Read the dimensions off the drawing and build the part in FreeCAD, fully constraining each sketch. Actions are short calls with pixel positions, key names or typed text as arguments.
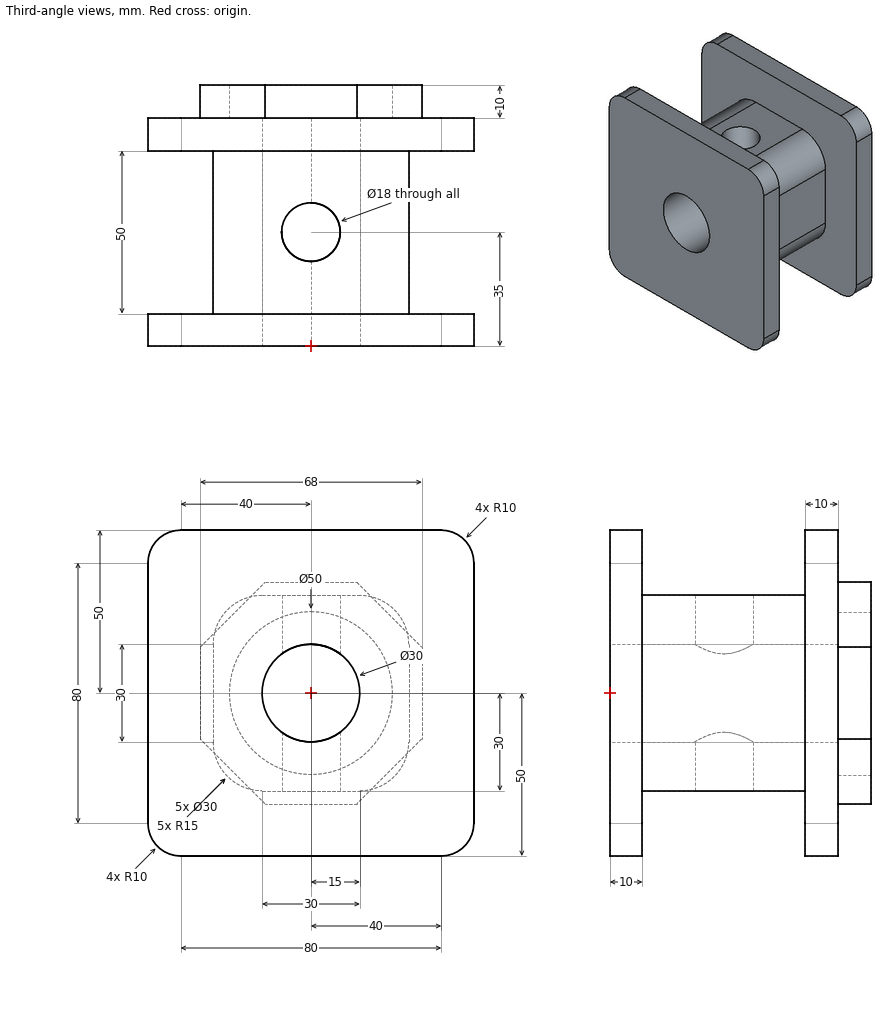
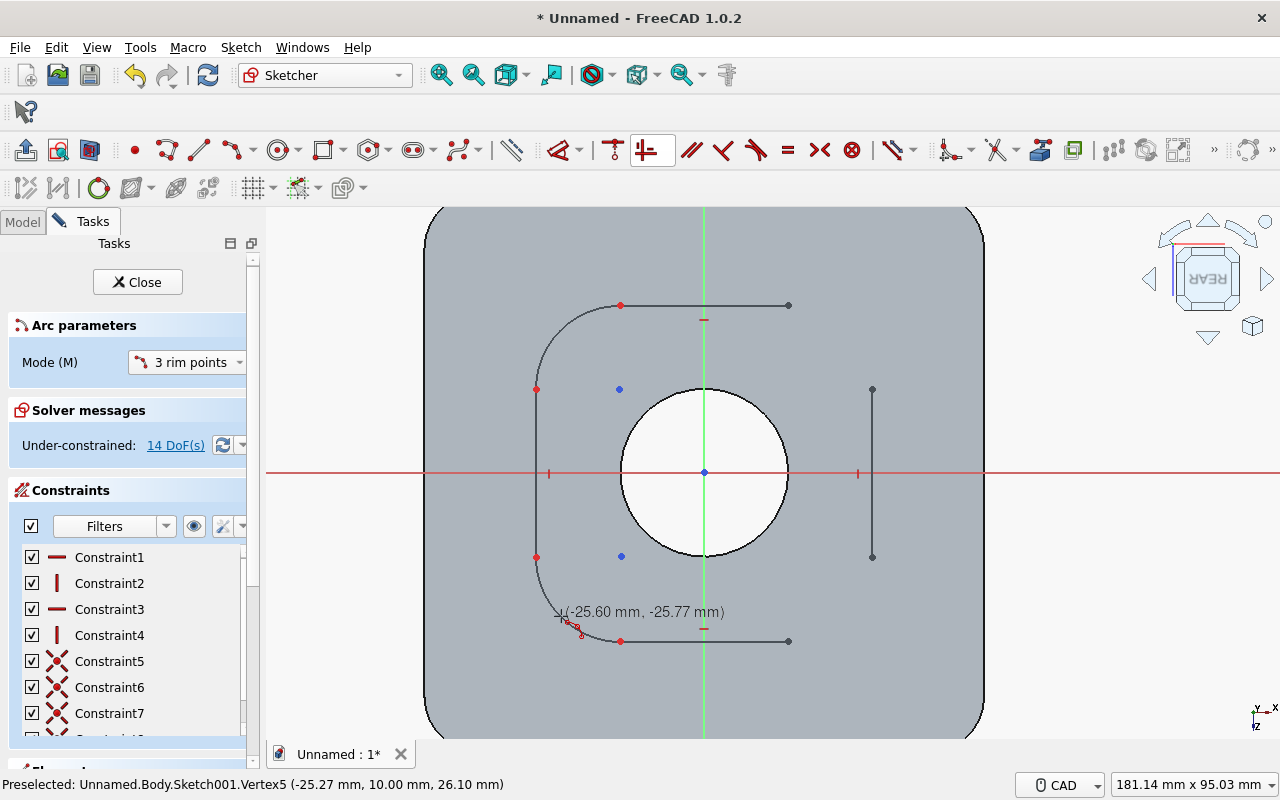
click(788, 642)
click(872, 558)
click(848, 616)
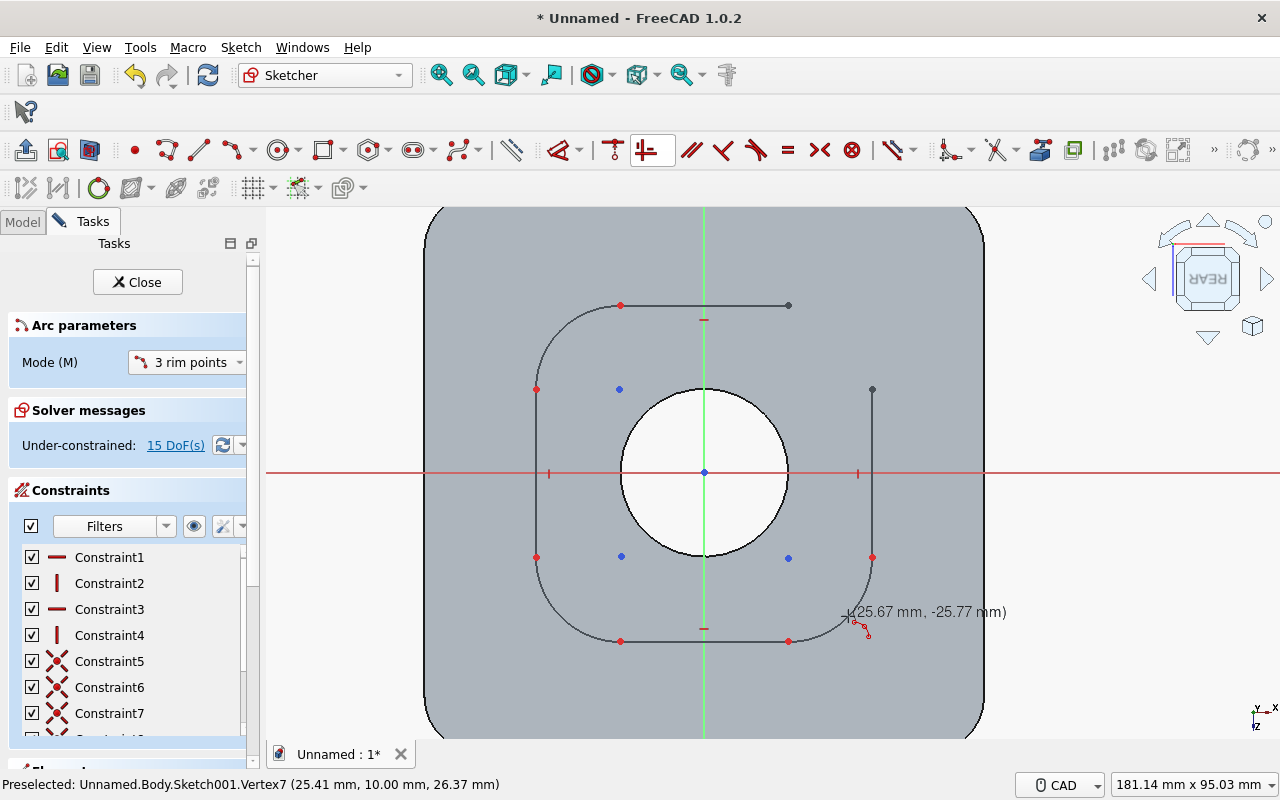
click(872, 390)
click(788, 306)
click(848, 329)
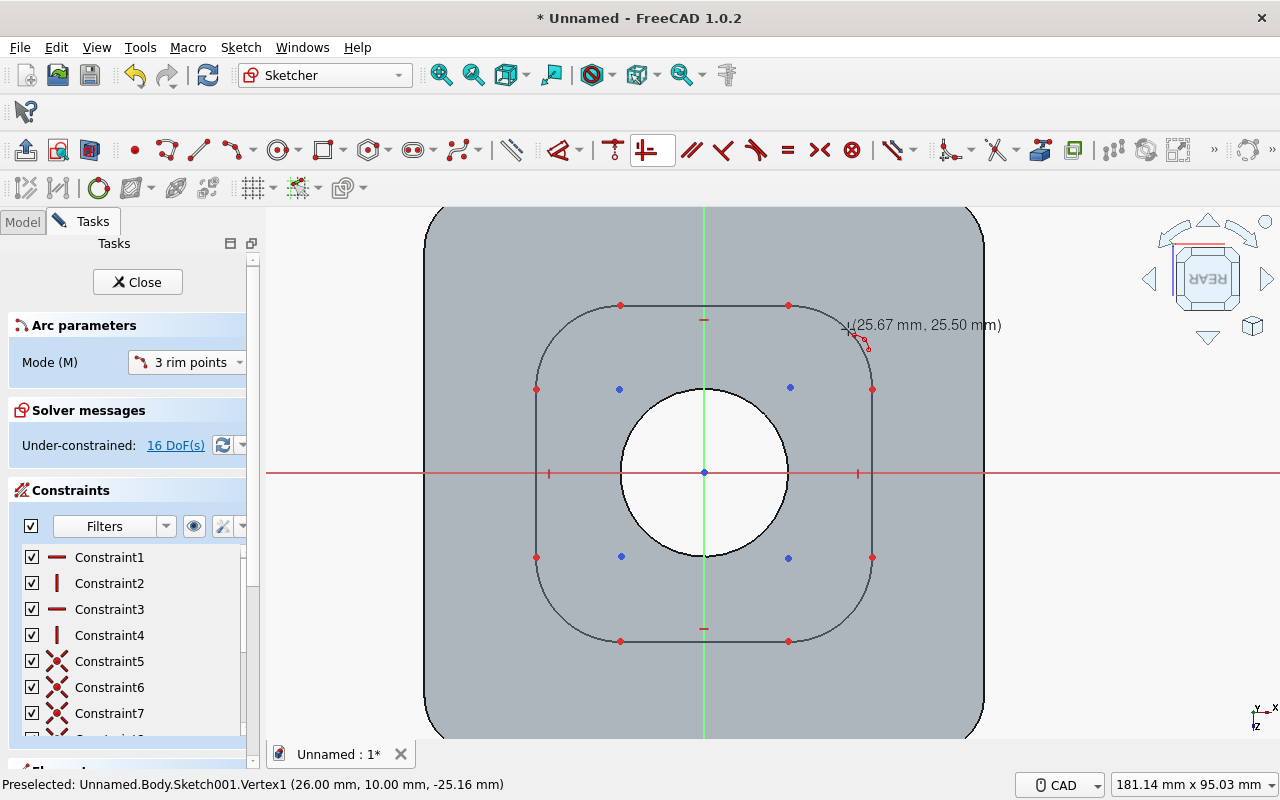
click(278, 150)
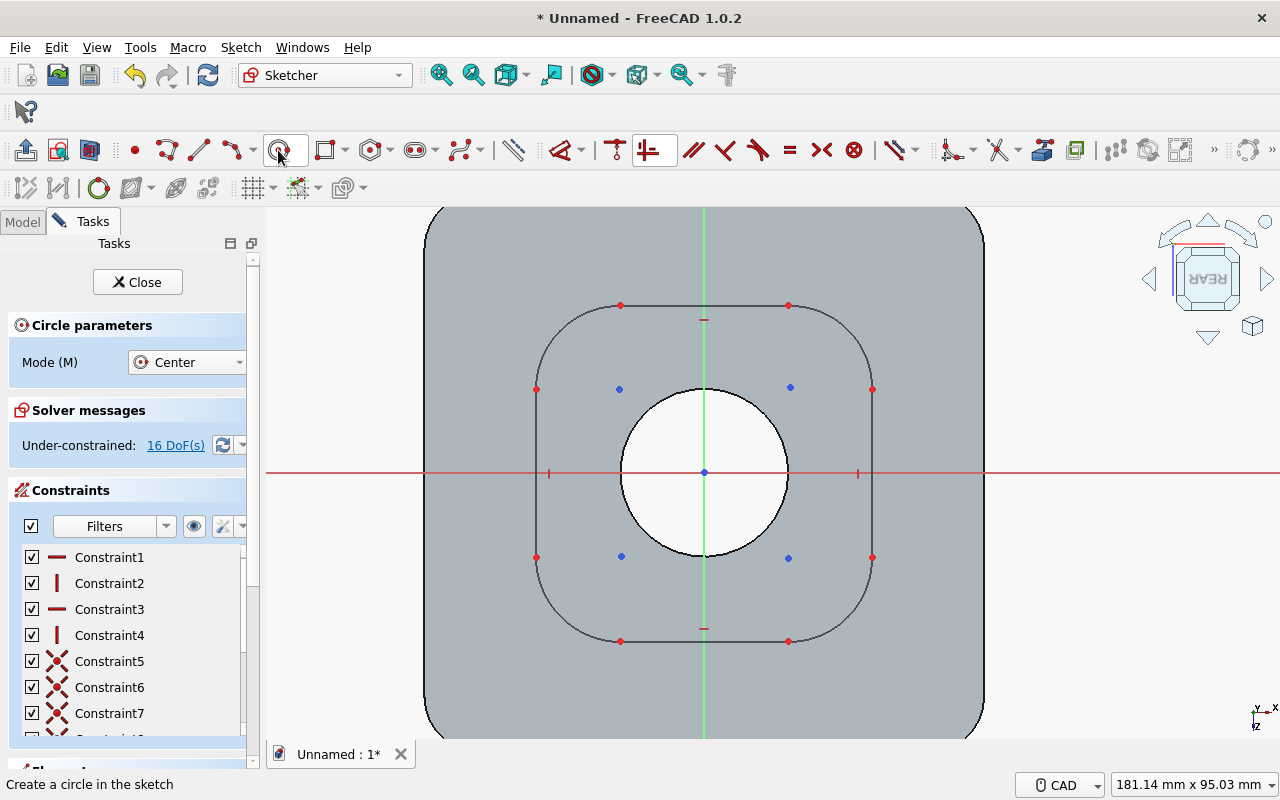
click(704, 473)
move(764, 413)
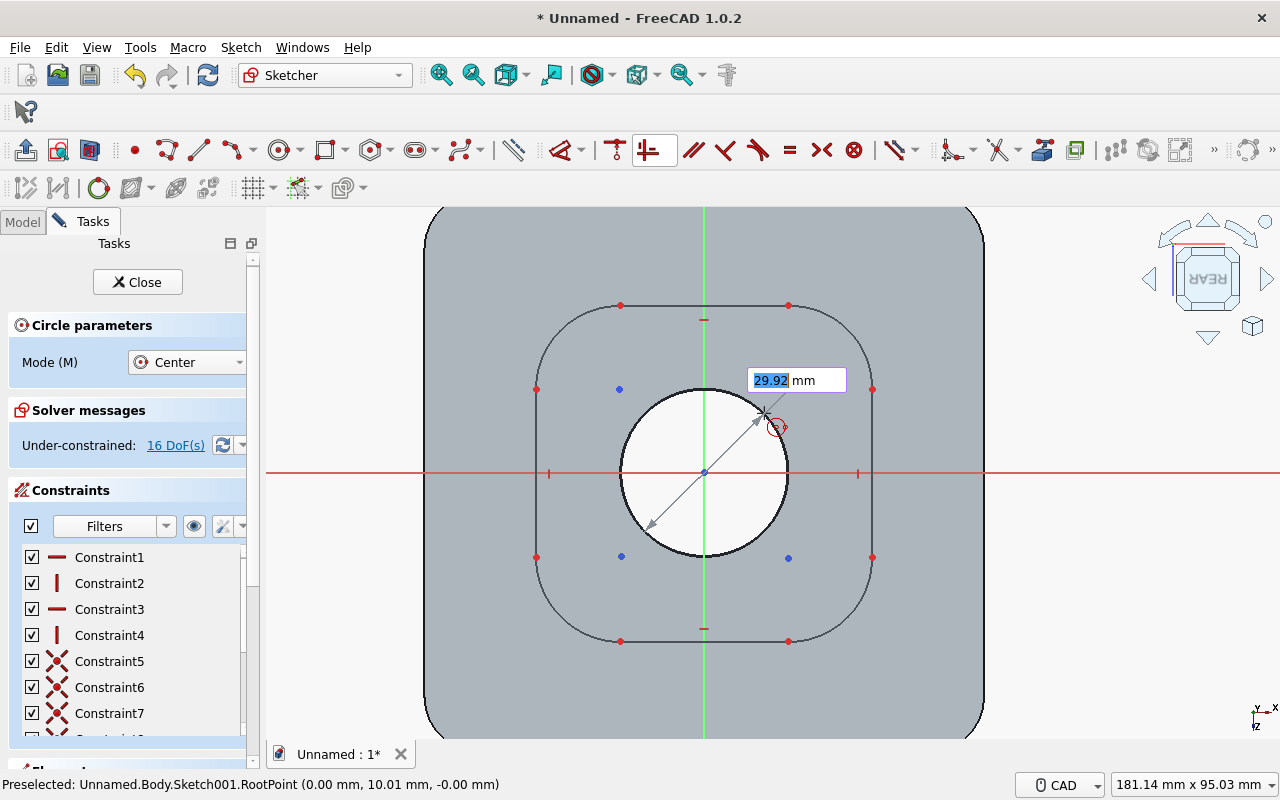
text(30)
key(Return)
key(Escape)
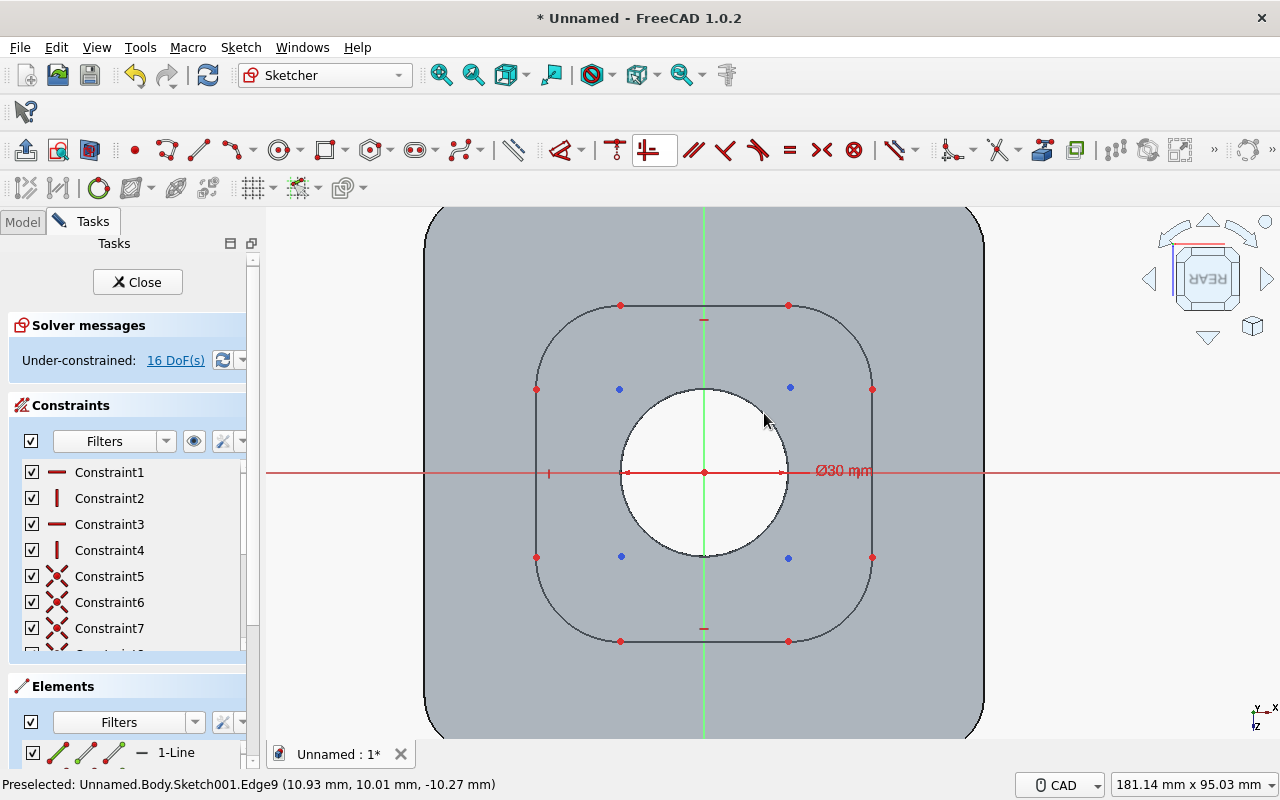
click(738, 306)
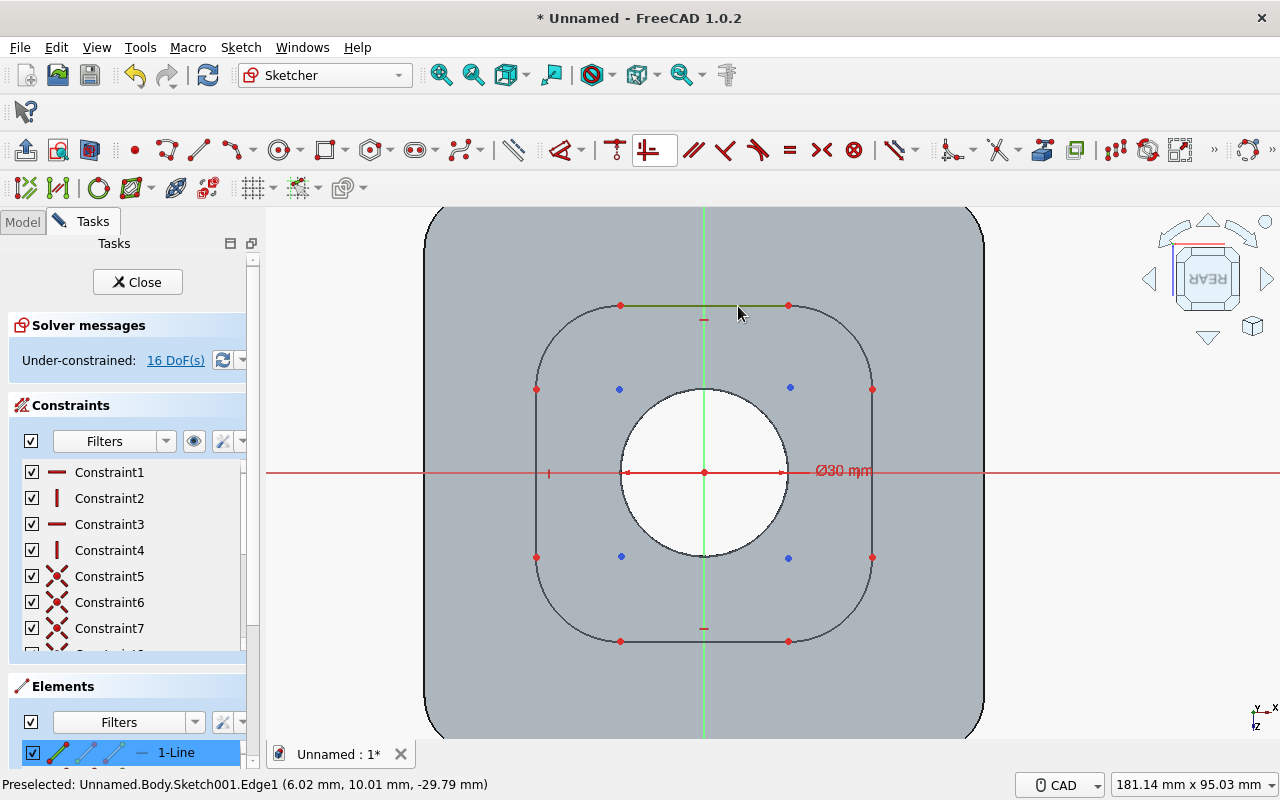
click(582, 315)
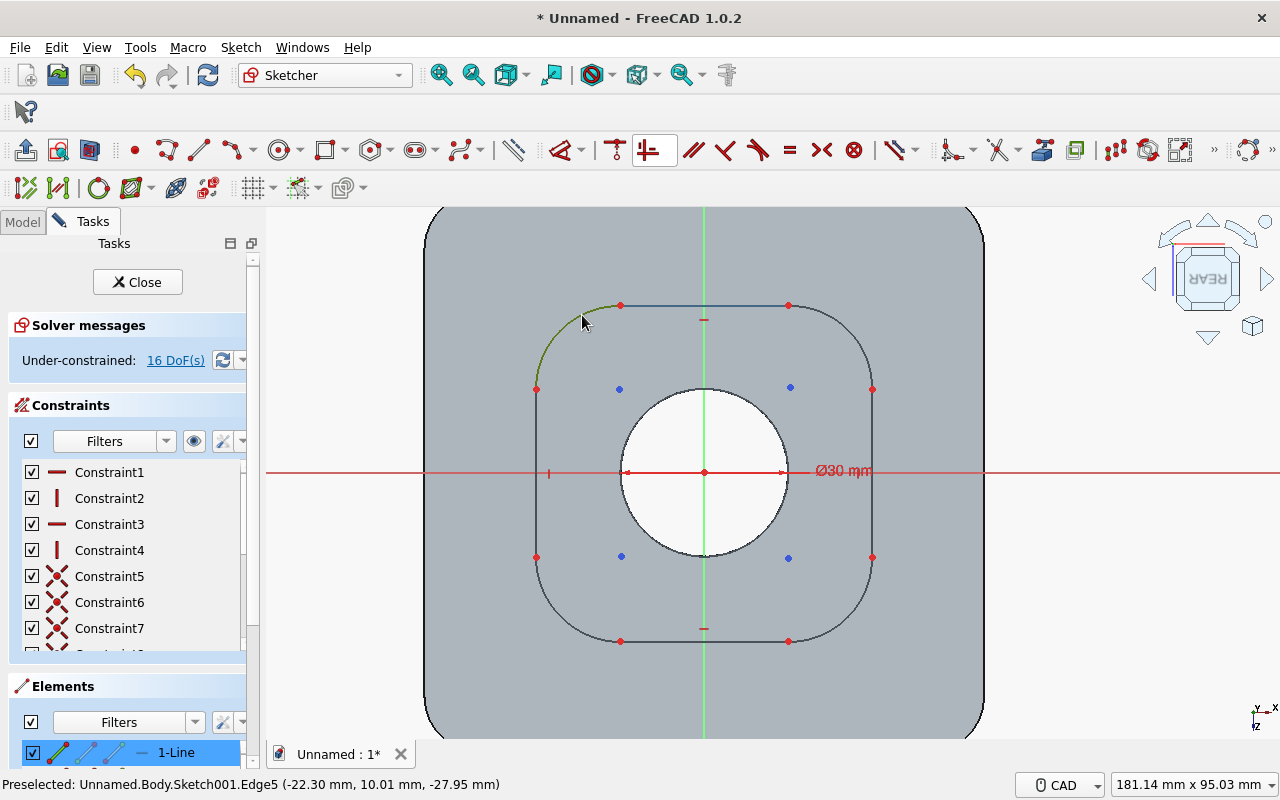
click(758, 150)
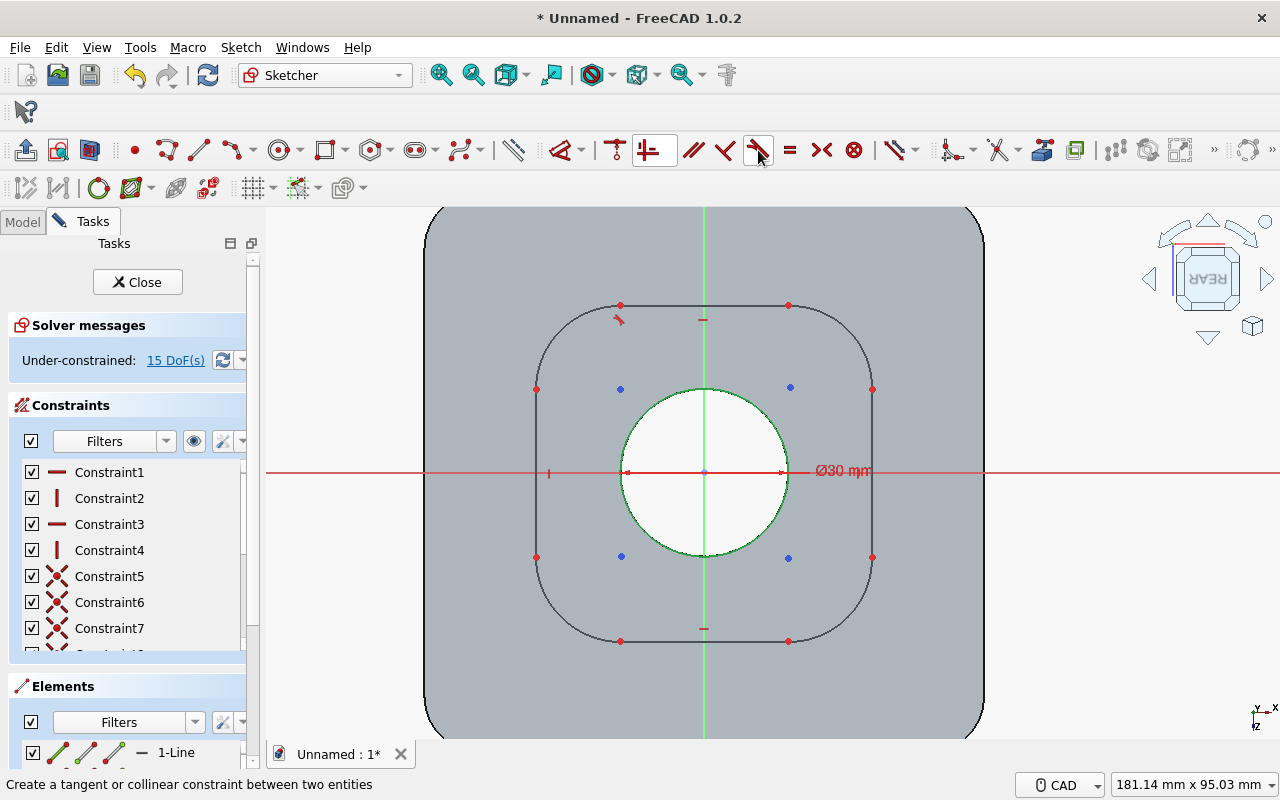
click(738, 306)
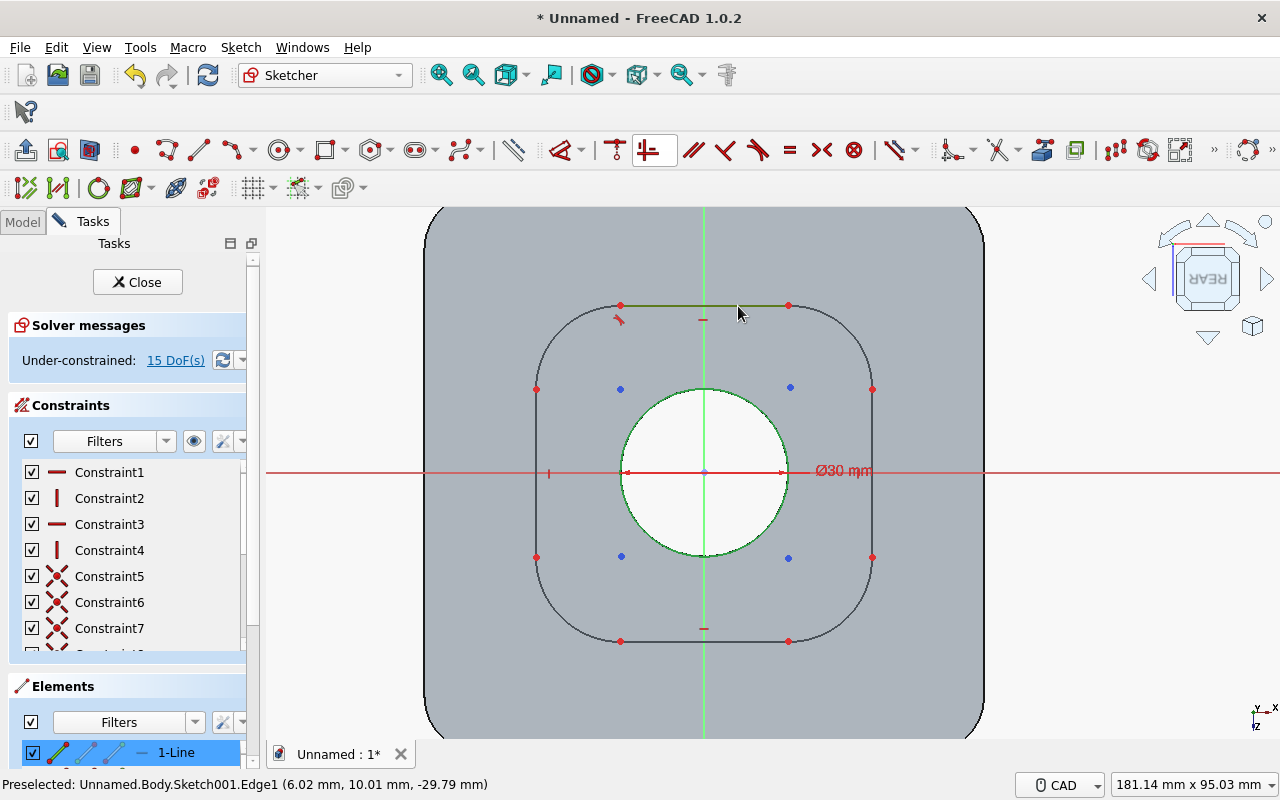
click(863, 351)